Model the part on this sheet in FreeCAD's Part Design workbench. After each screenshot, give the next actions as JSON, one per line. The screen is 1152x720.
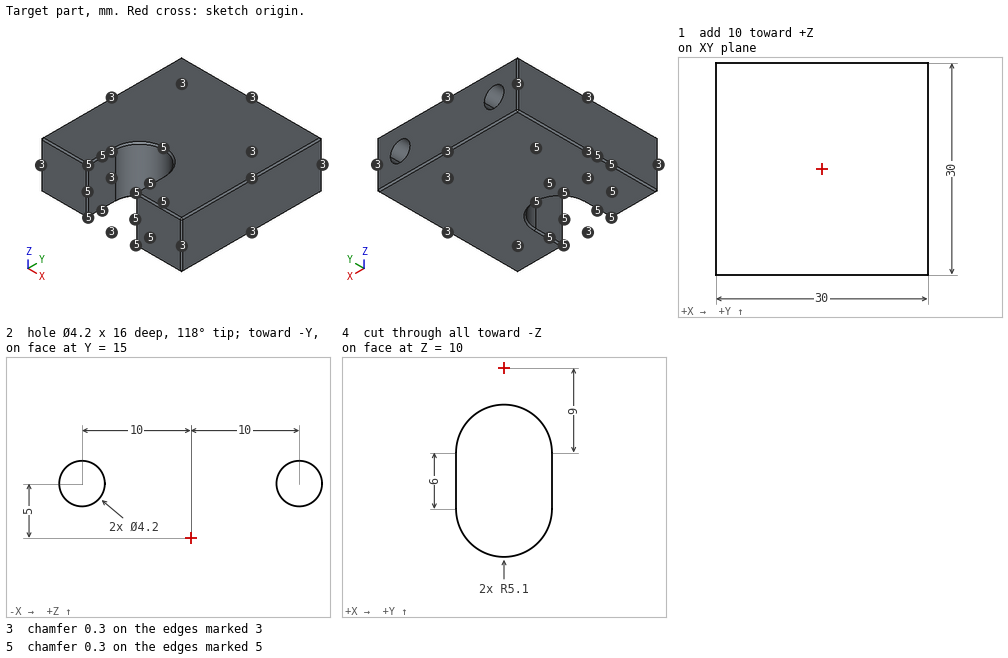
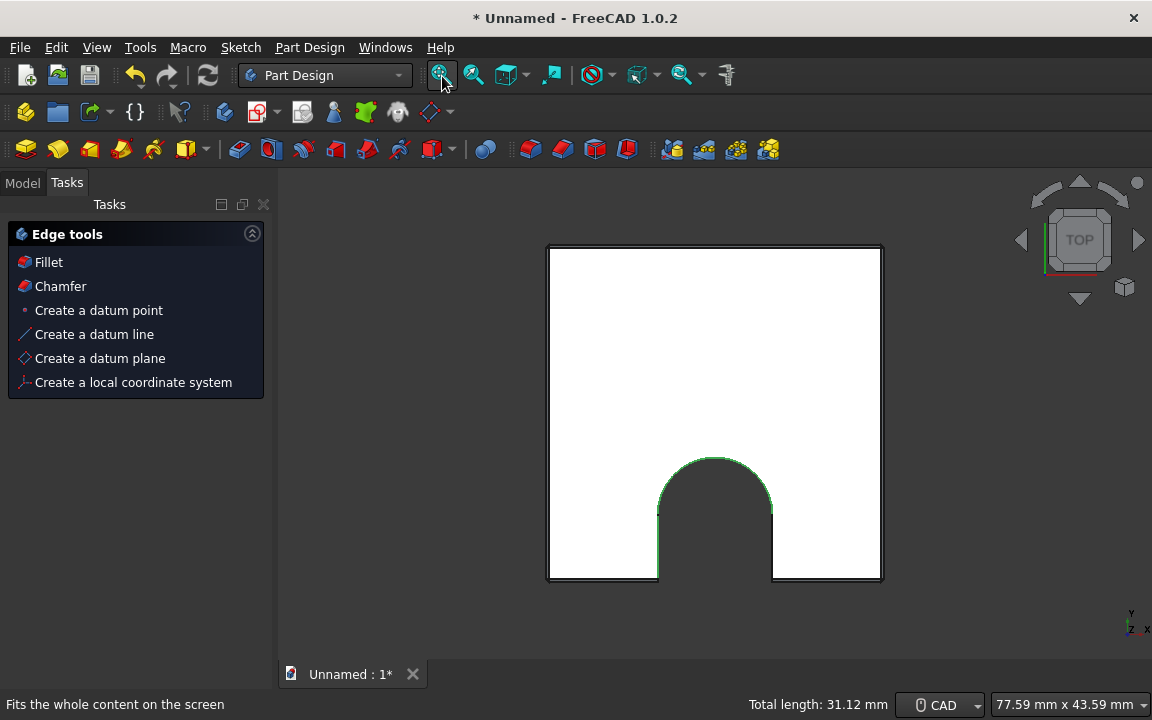
{"action": "left_click", "coordinate": [772, 546], "text": "ctrl"}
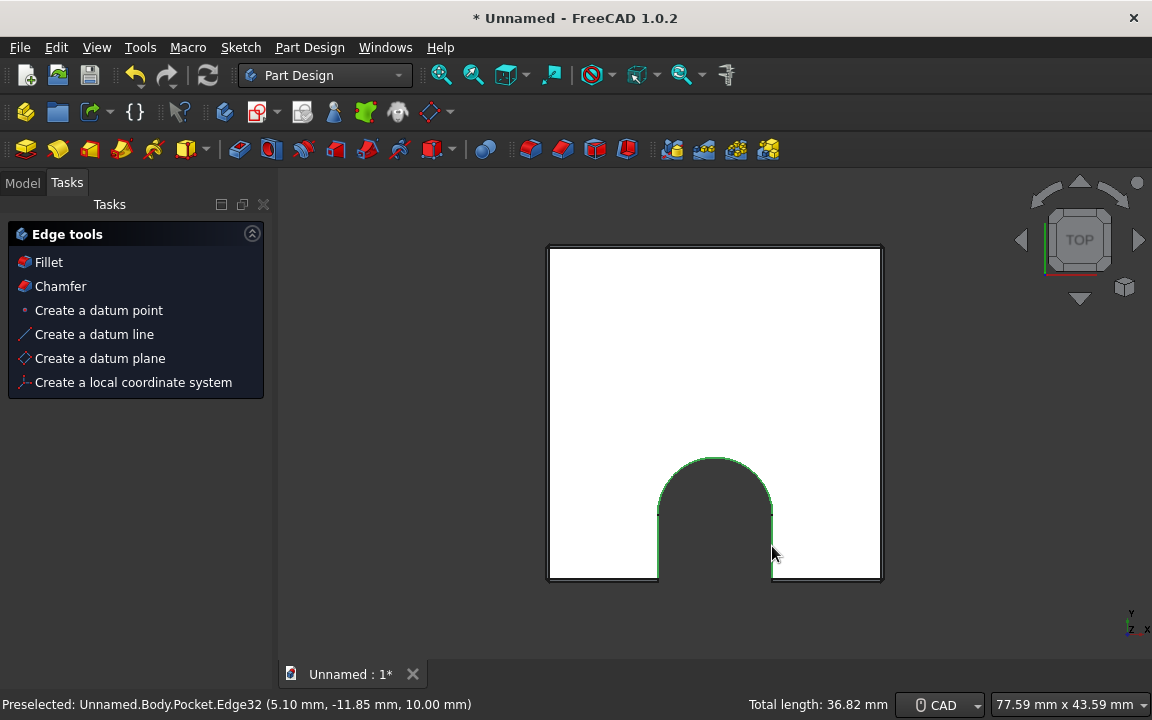
{"action": "scroll", "coordinate": [772, 580], "scroll_direction": "up", "scroll_amount": 11}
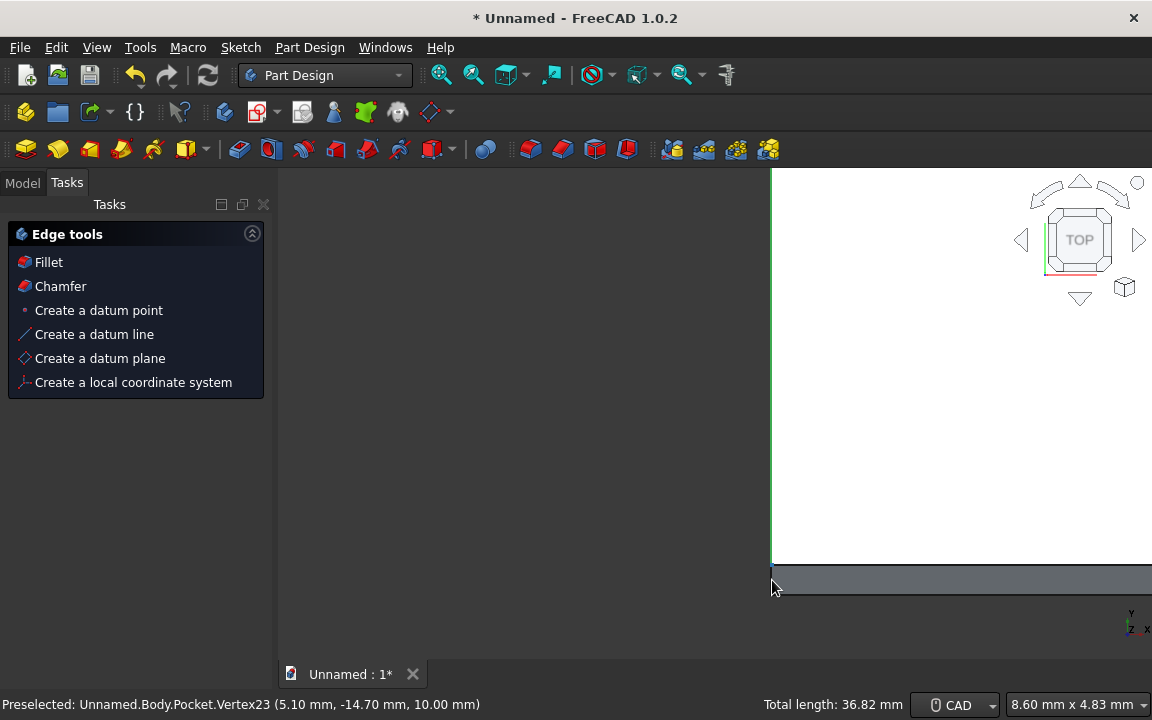
{"action": "left_click", "coordinate": [772, 579], "text": "ctrl"}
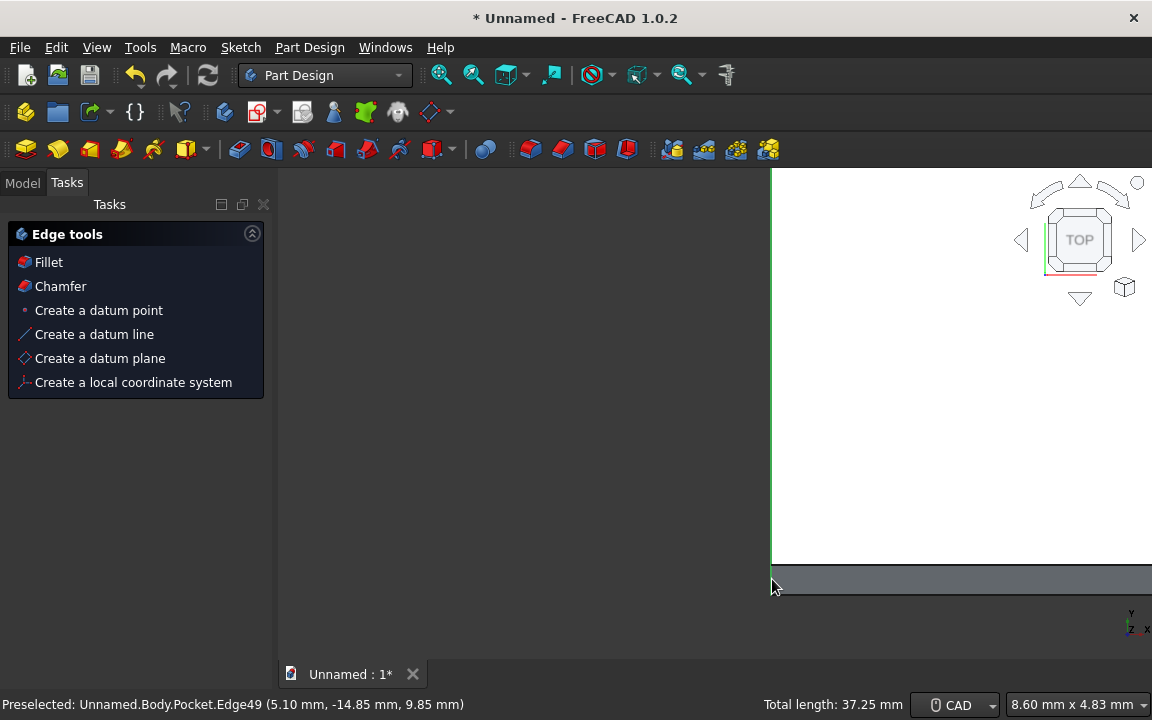
{"action": "left_click", "coordinate": [442, 76]}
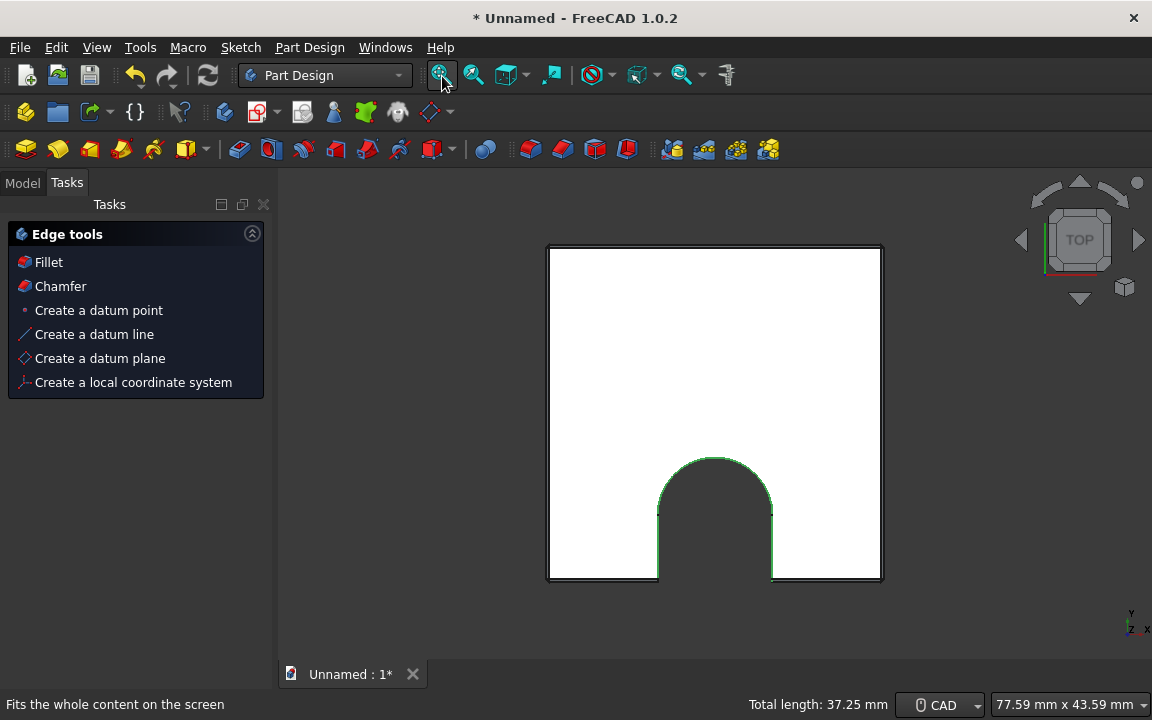
{"action": "key", "text": "0"}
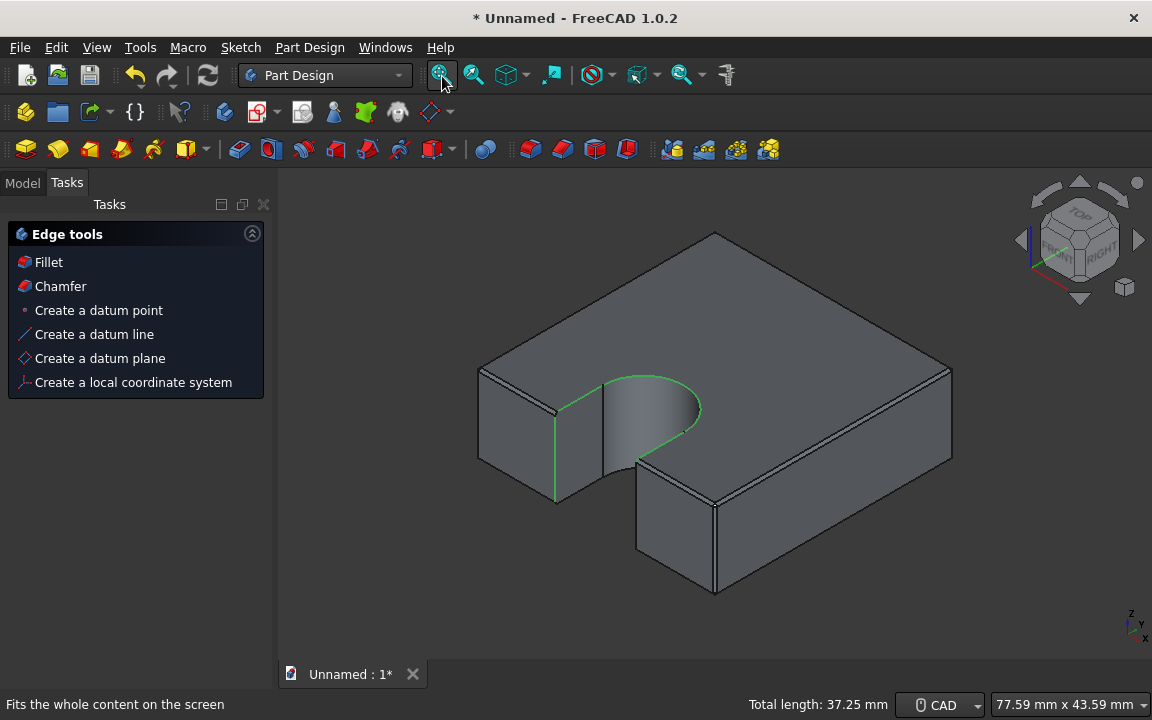
{"action": "scroll", "coordinate": [637, 549], "scroll_direction": "up", "scroll_amount": 11}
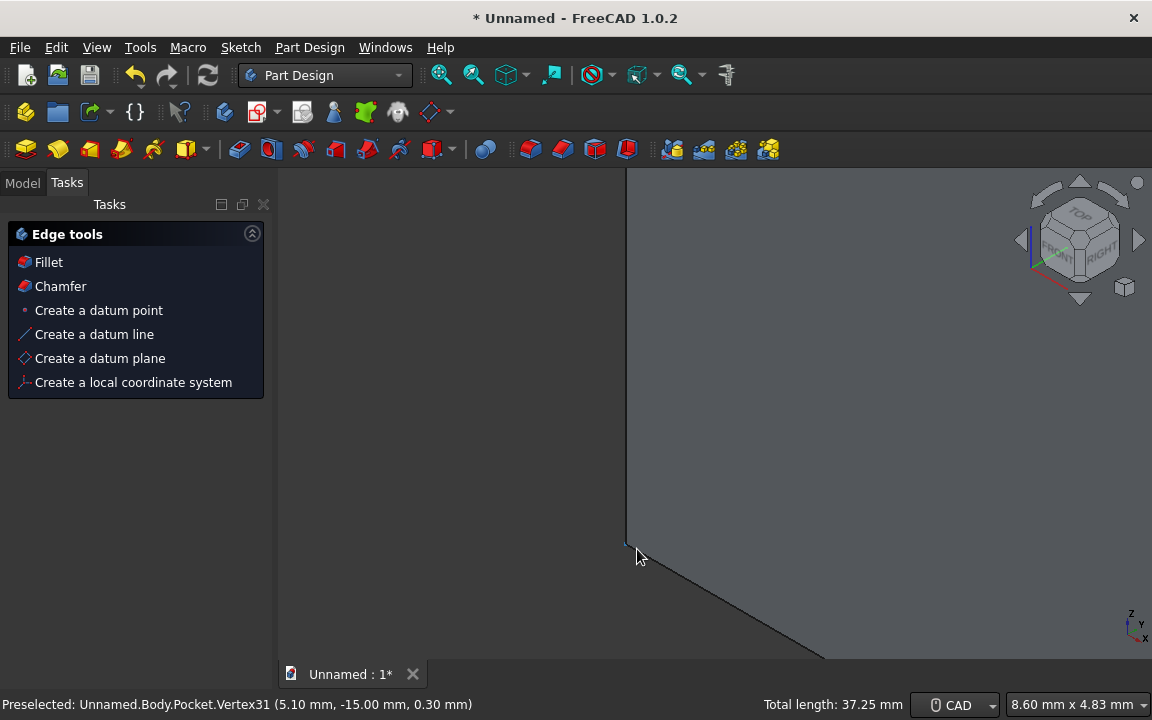
{"action": "left_click", "coordinate": [442, 76]}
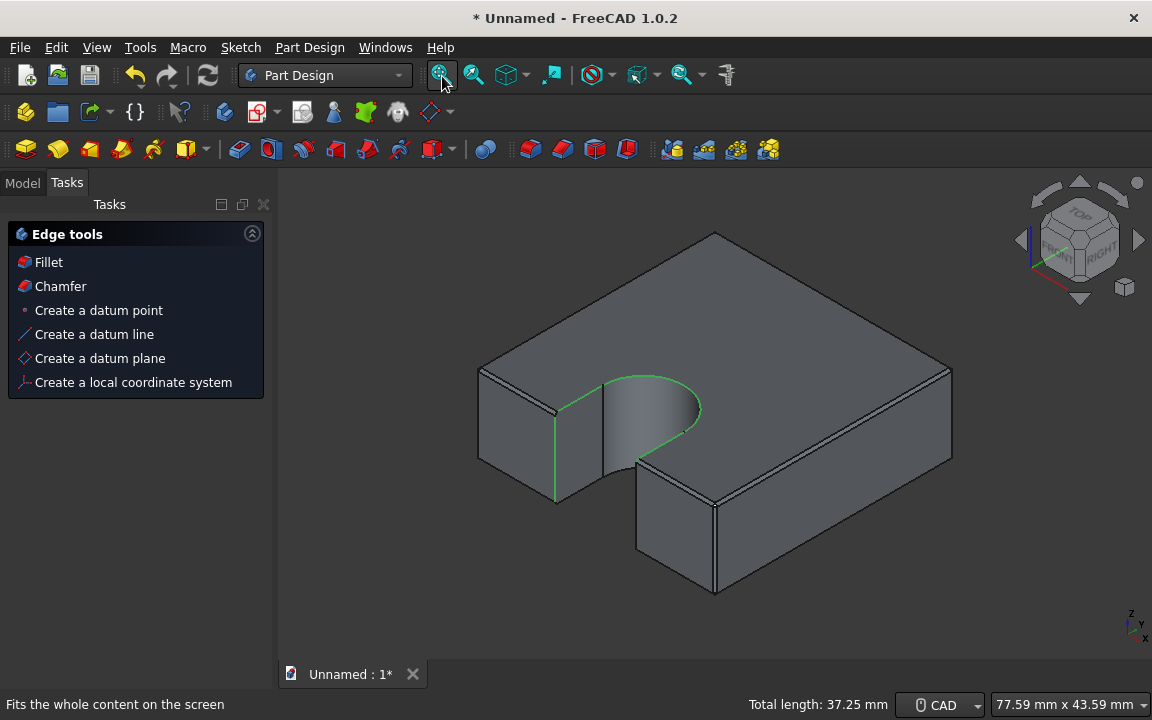
{"action": "key", "text": "1"}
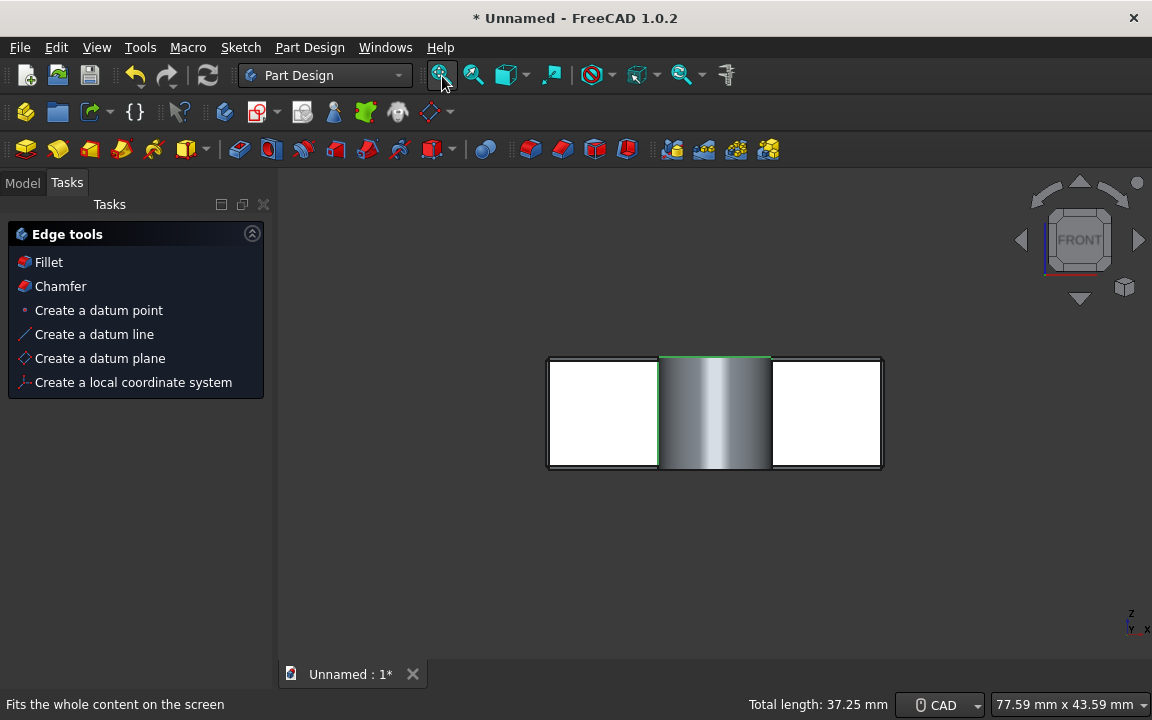
{"action": "left_click", "coordinate": [442, 76]}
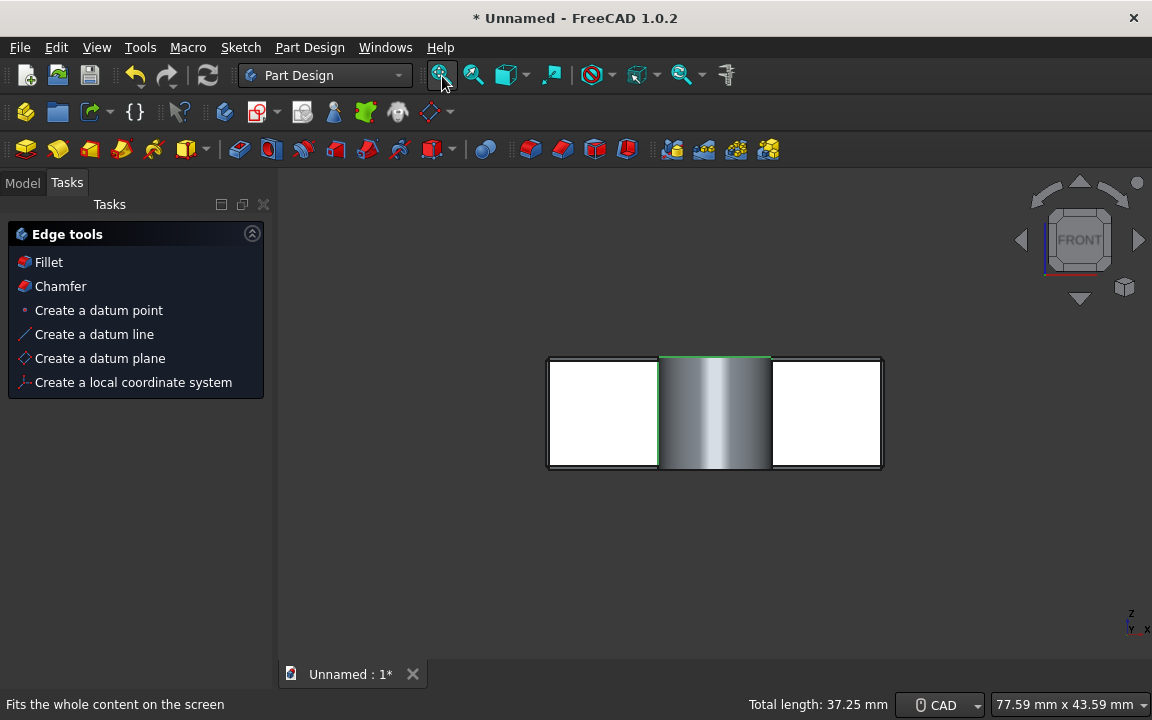
{"action": "left_click", "coordinate": [772, 413], "text": "ctrl"}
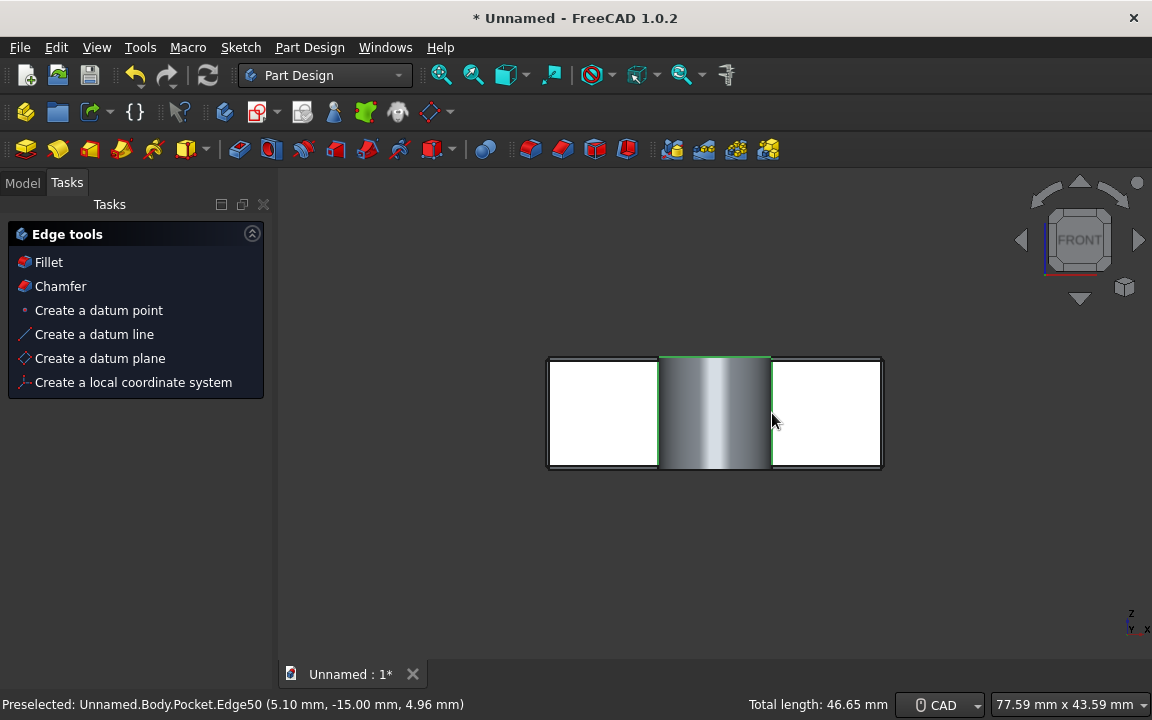
{"action": "left_click", "coordinate": [715, 469], "text": "ctrl"}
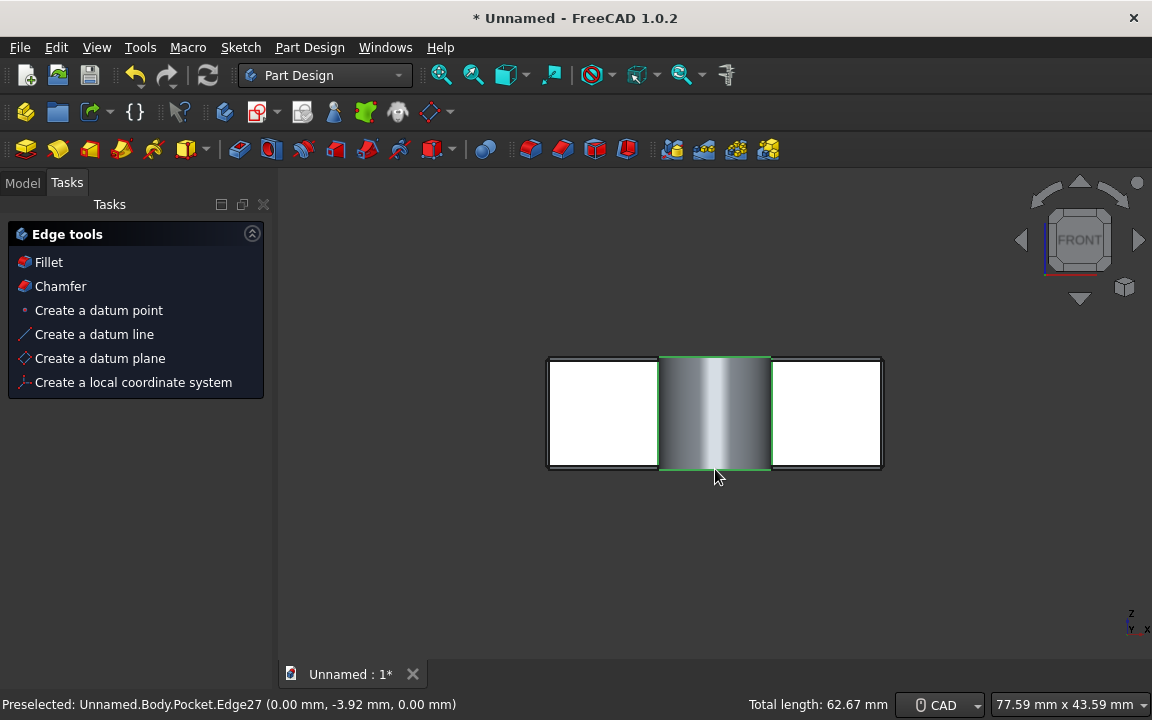
{"action": "scroll", "coordinate": [772, 467], "scroll_direction": "up", "scroll_amount": 11}